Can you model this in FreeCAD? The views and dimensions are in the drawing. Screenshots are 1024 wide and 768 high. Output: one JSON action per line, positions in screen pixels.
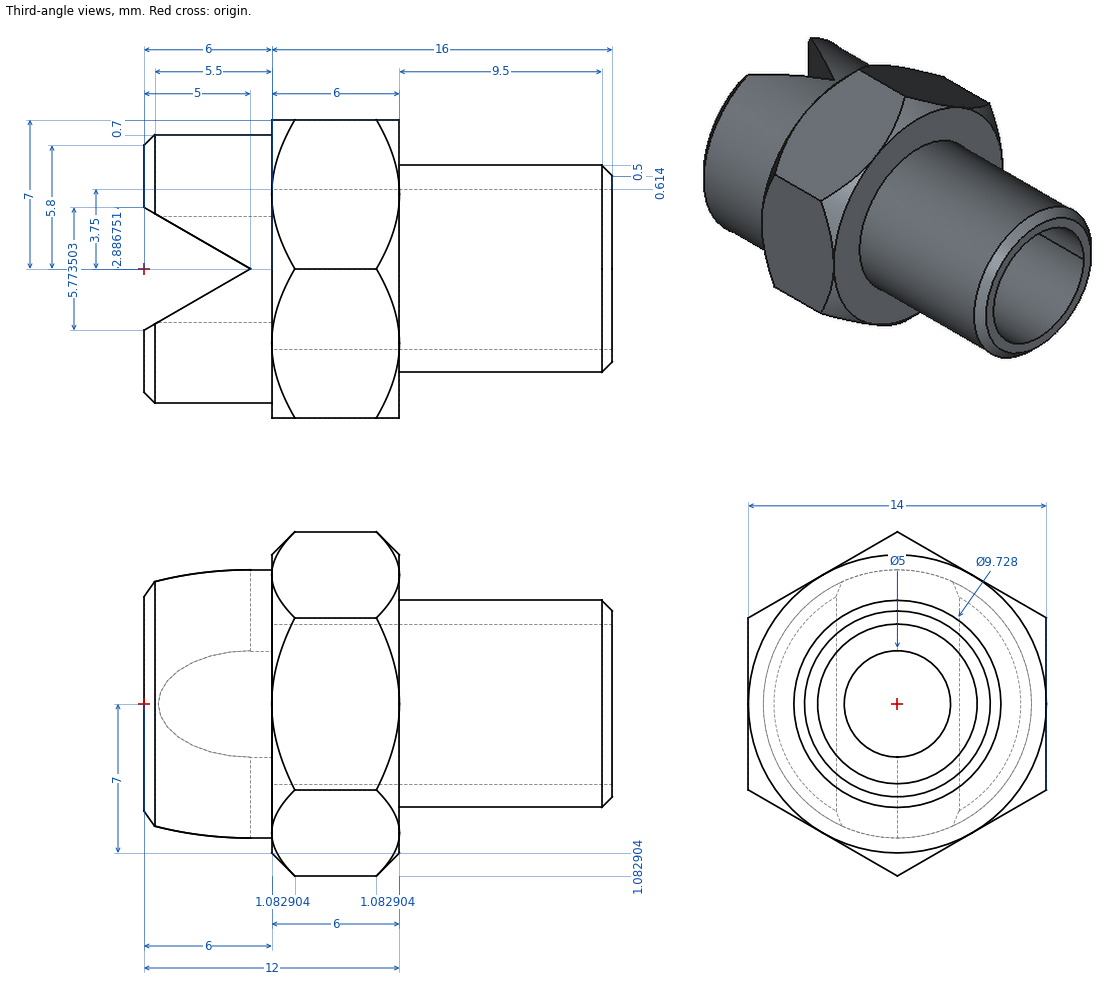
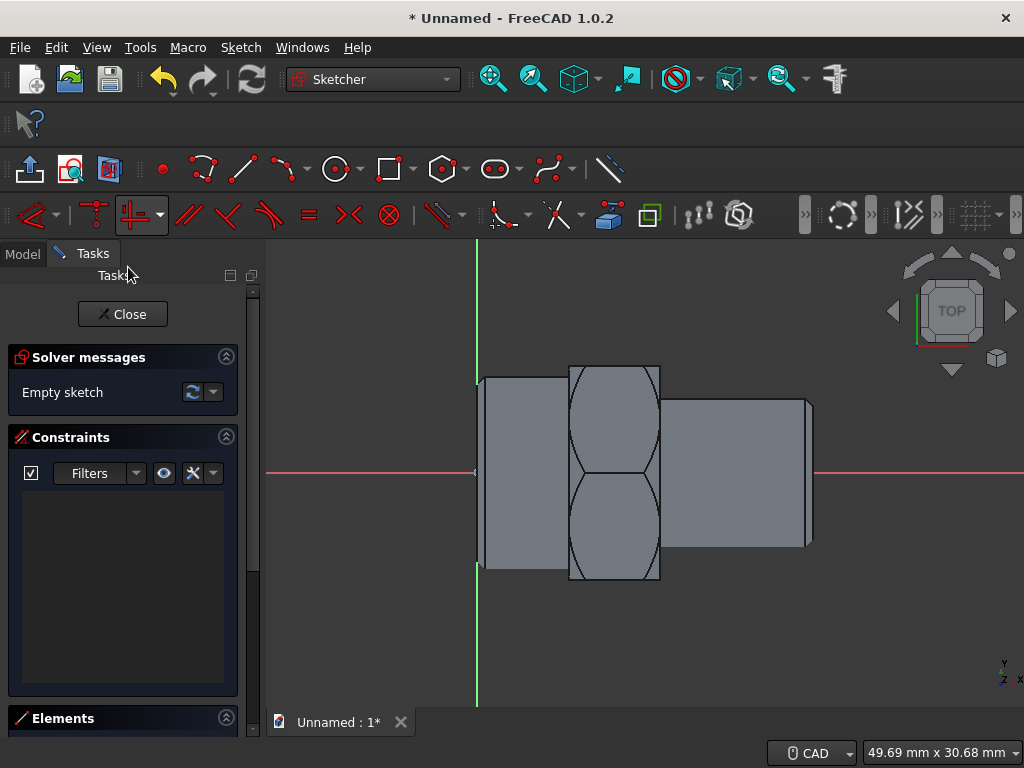
{"action": "left_click", "coordinate": [110, 170]}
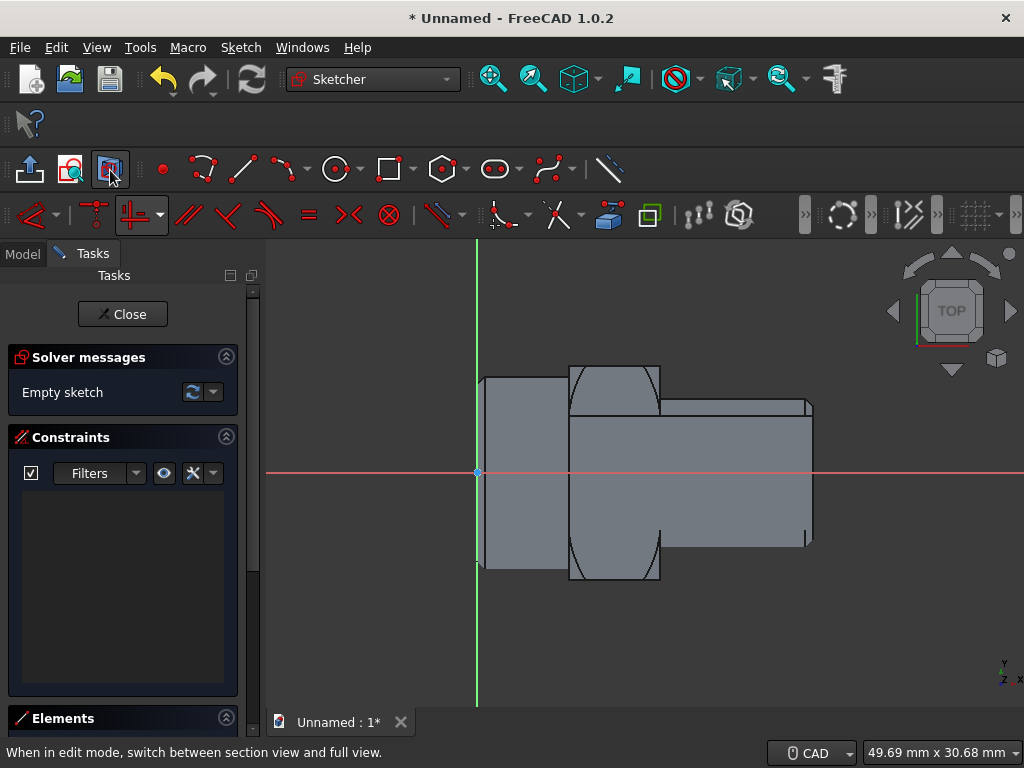
{"action": "scroll", "coordinate": [489, 473], "scroll_direction": "up", "scroll_amount": 6}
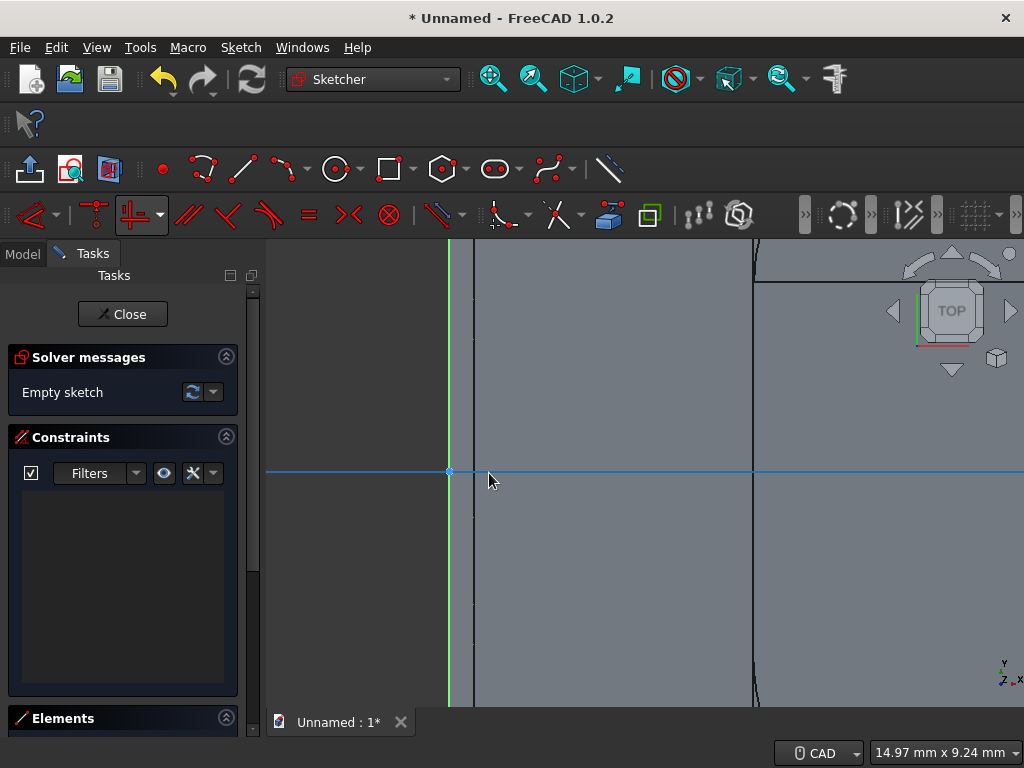
{"action": "left_click", "coordinate": [204, 170]}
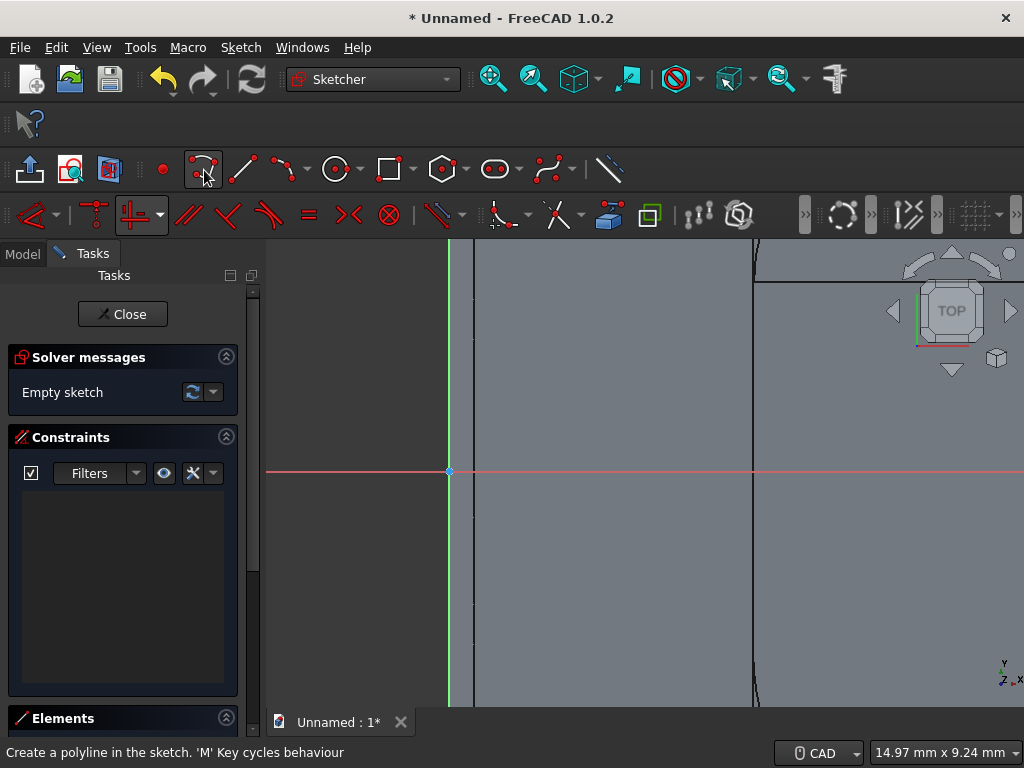
{"action": "left_click", "coordinate": [449, 326]}
{"action": "left_click", "coordinate": [458, 618]}
{"action": "left_click", "coordinate": [702, 472]}
{"action": "left_click", "coordinate": [449, 327]}
{"action": "key", "text": "Escape"}
{"action": "key", "text": "Escape"}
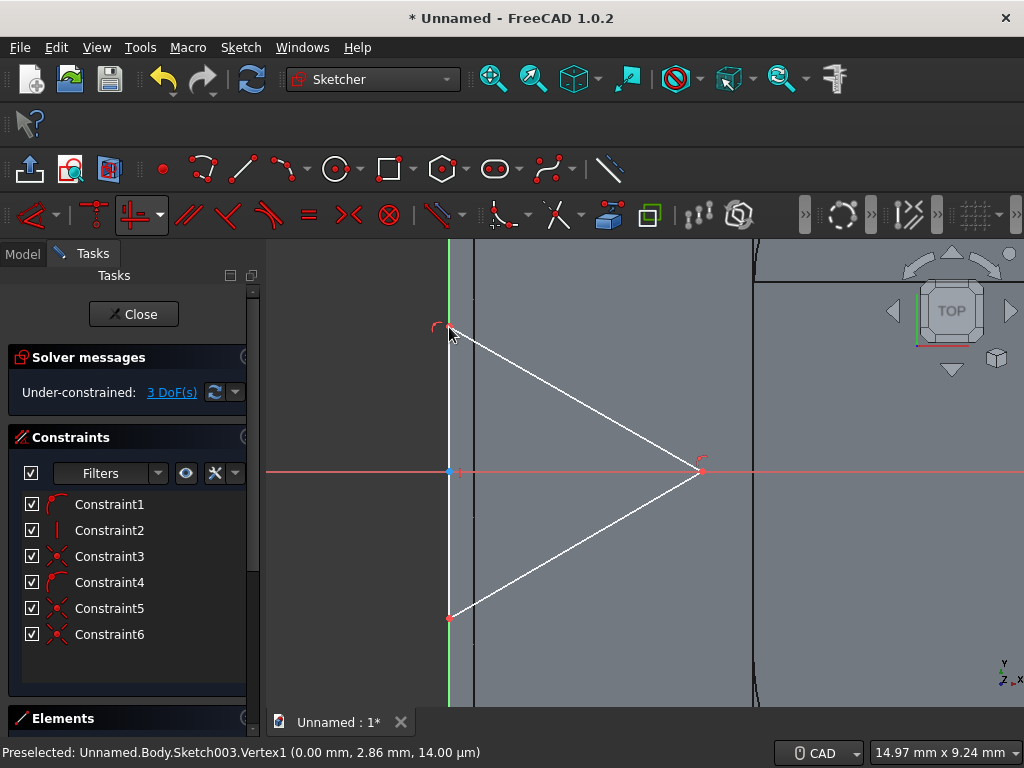
{"action": "left_click", "coordinate": [32, 216]}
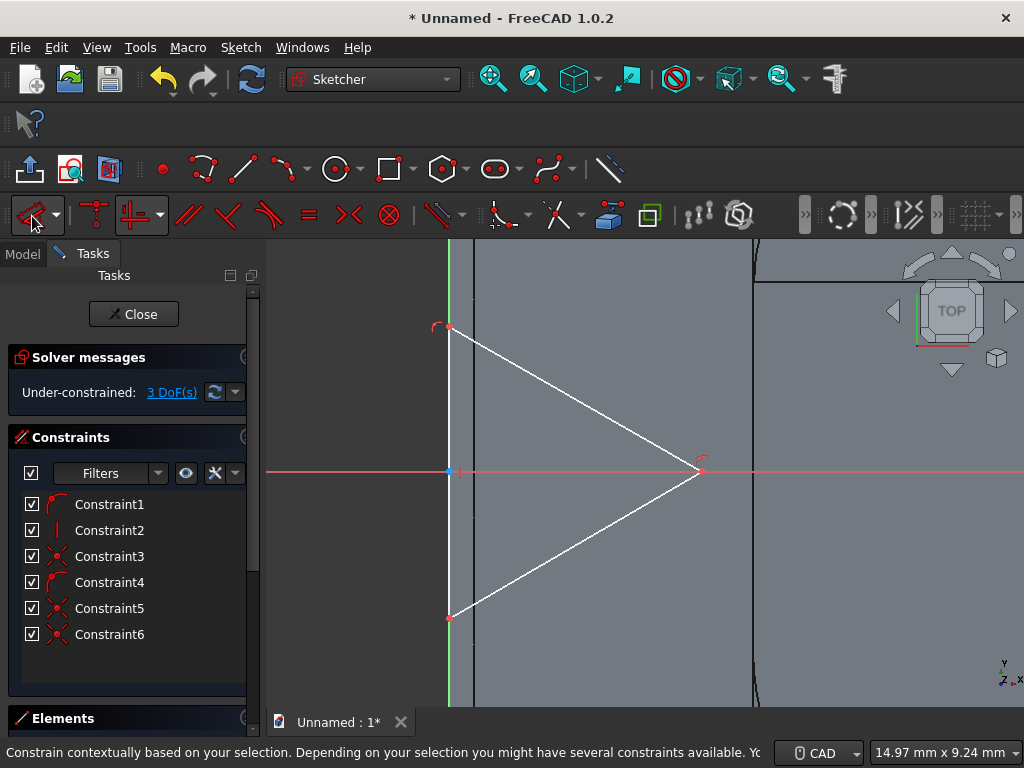
{"action": "left_click", "coordinate": [702, 472]}
{"action": "left_click", "coordinate": [576, 506]}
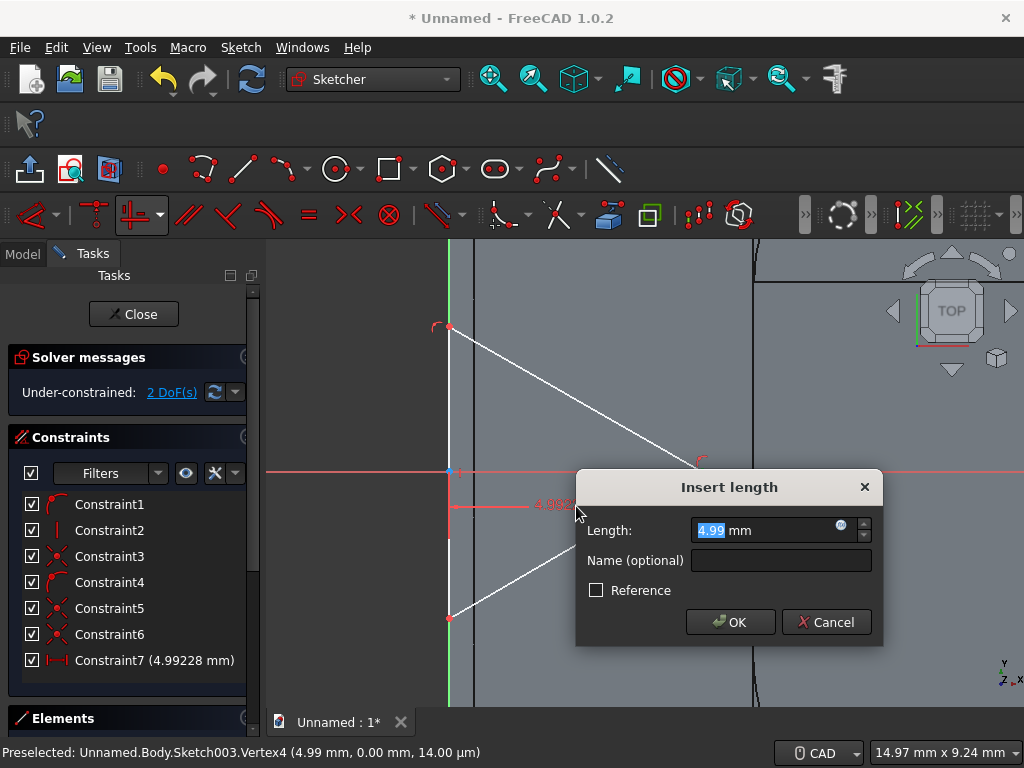
{"action": "type", "text": "5"}
{"action": "key", "text": "Return"}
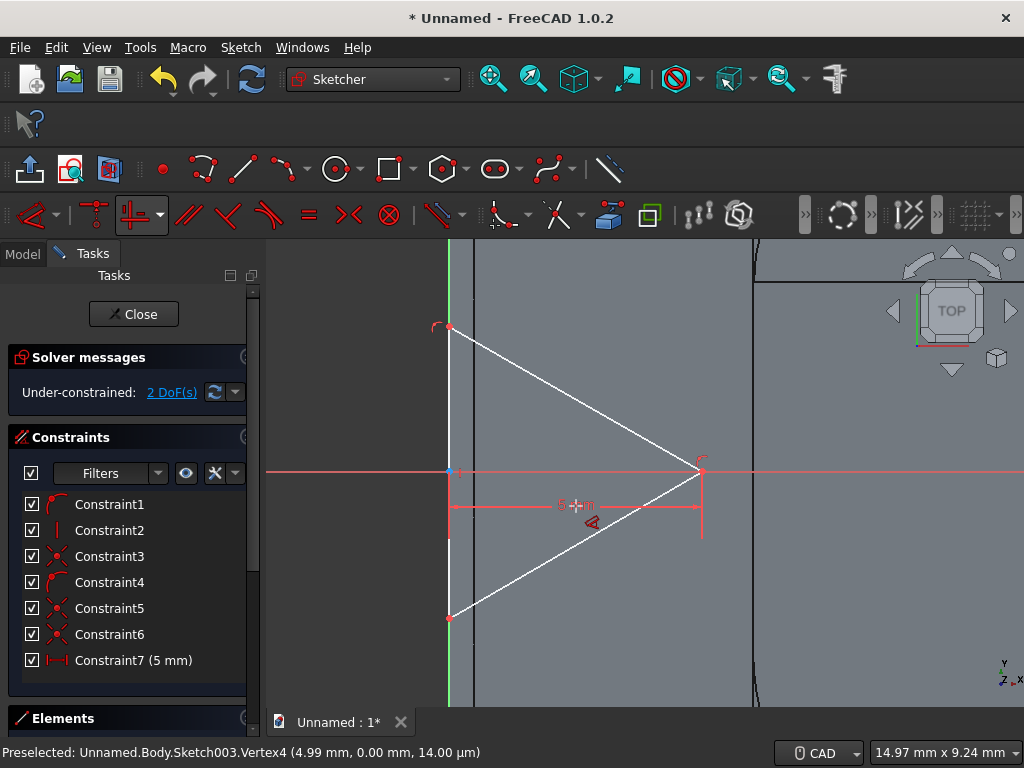
{"action": "left_click", "coordinate": [449, 415]}
{"action": "left_click", "coordinate": [415, 406]}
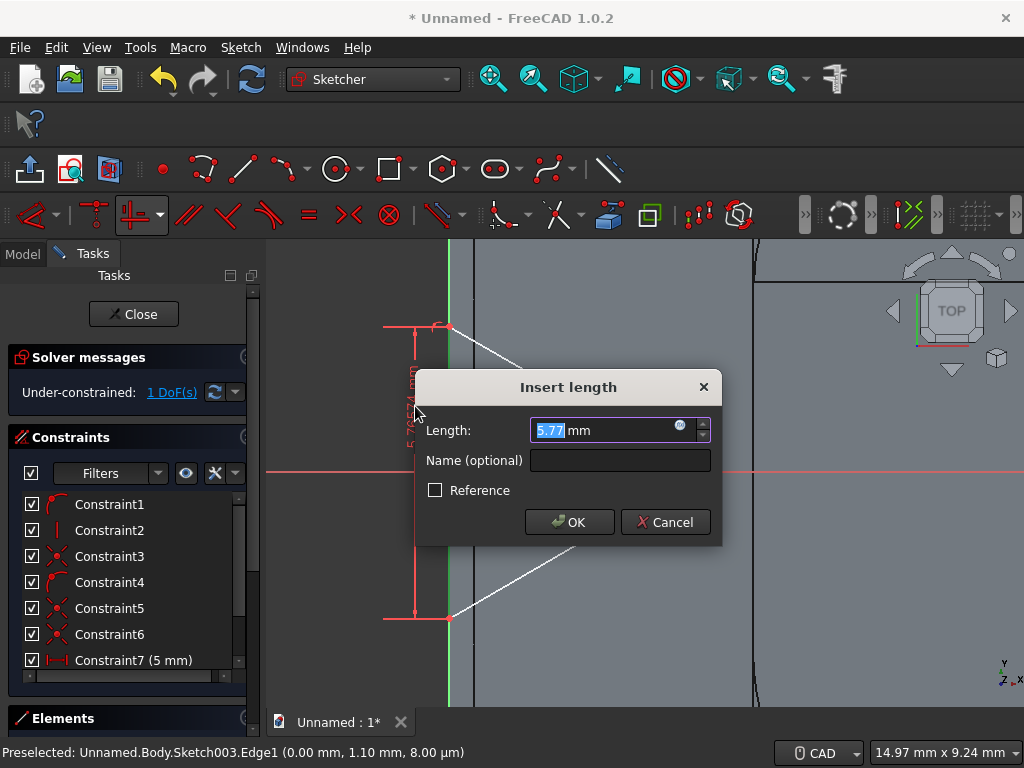
{"action": "type", "text": "5.773503"}
{"action": "key", "text": "Return"}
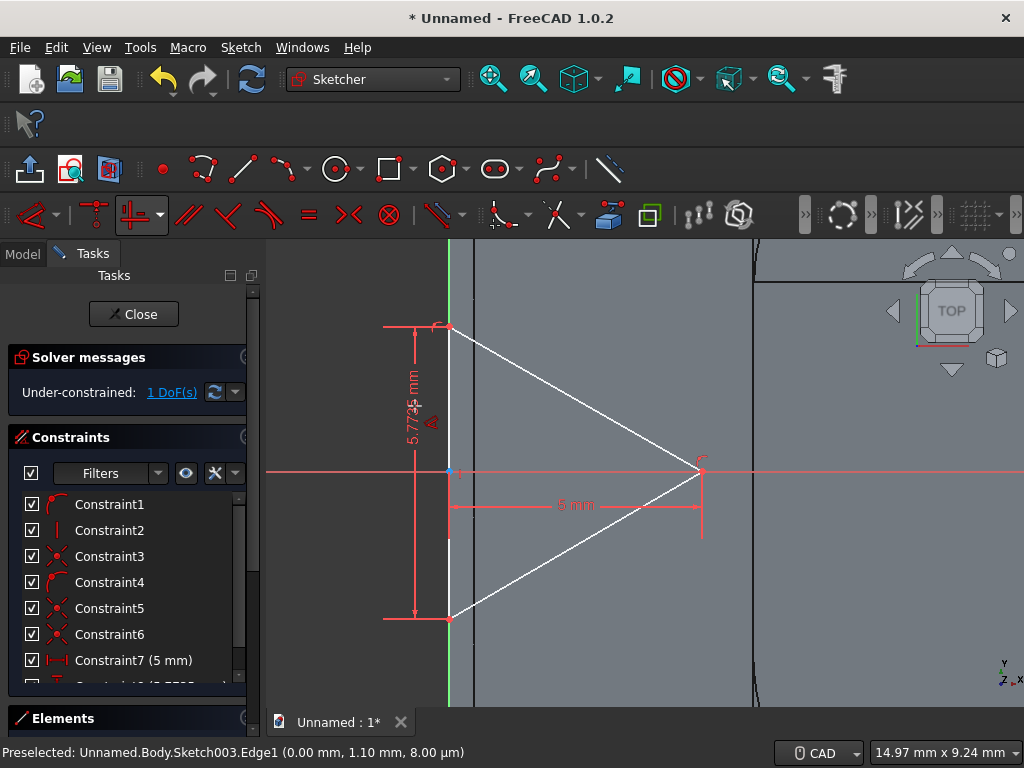
{"action": "left_click", "coordinate": [449, 327]}
{"action": "left_click", "coordinate": [415, 366]}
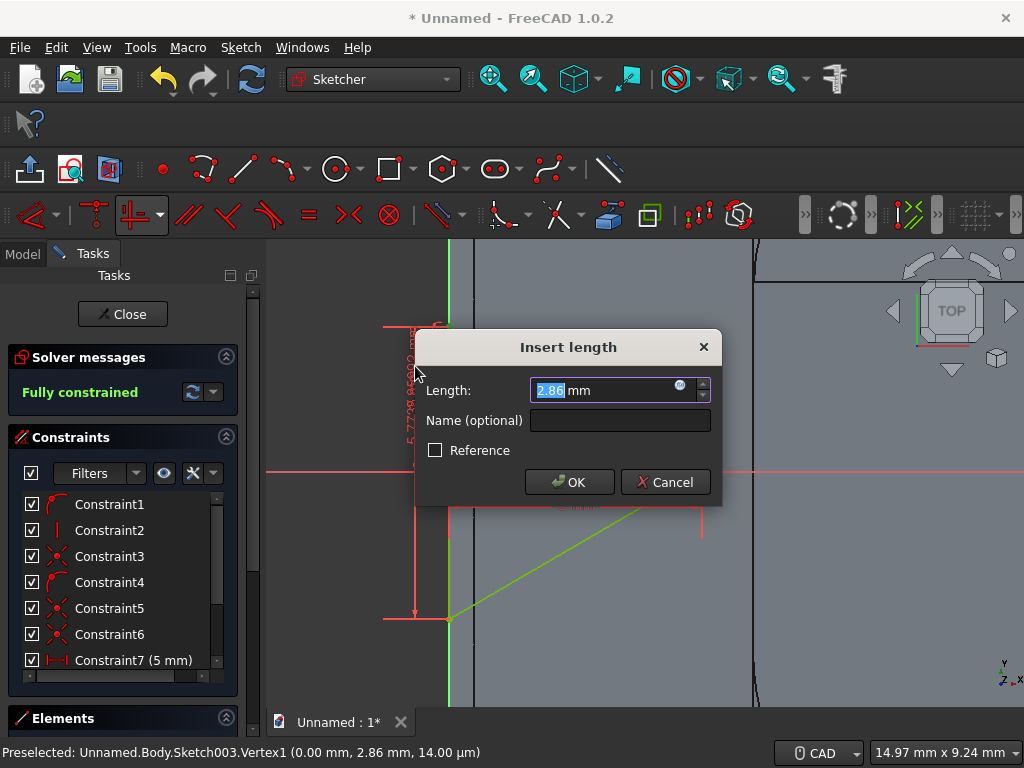
{"action": "type", "text": "2.886751"}
{"action": "key", "text": "Return"}
{"action": "key", "text": "Escape"}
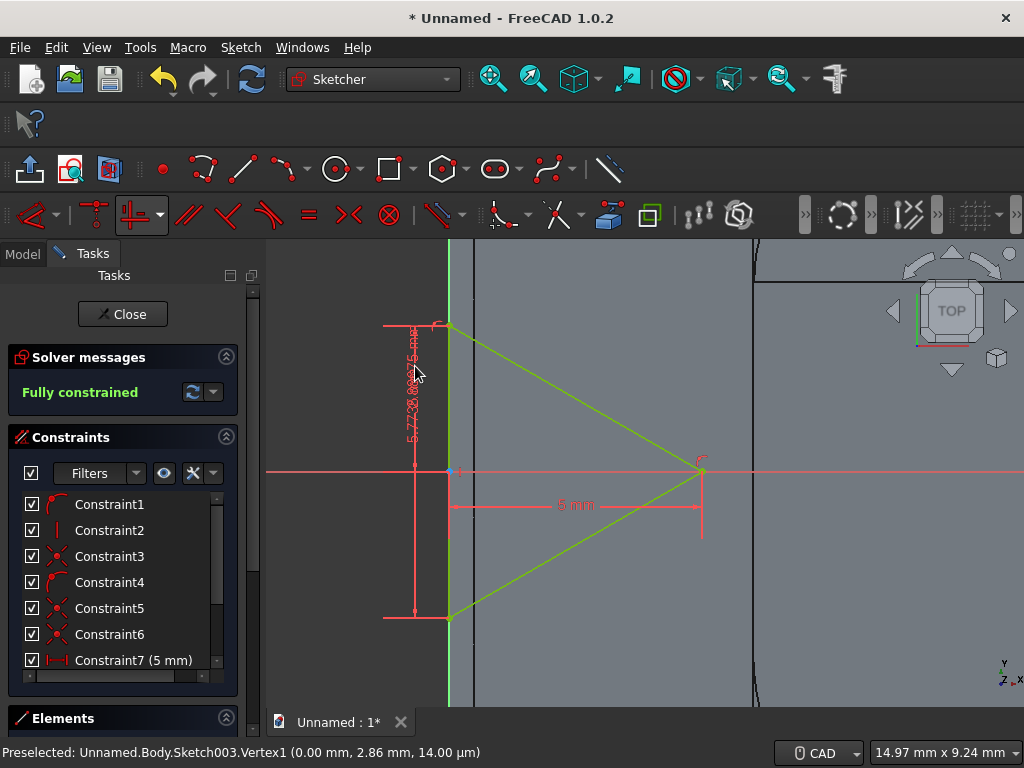
{"action": "left_click", "coordinate": [123, 314]}